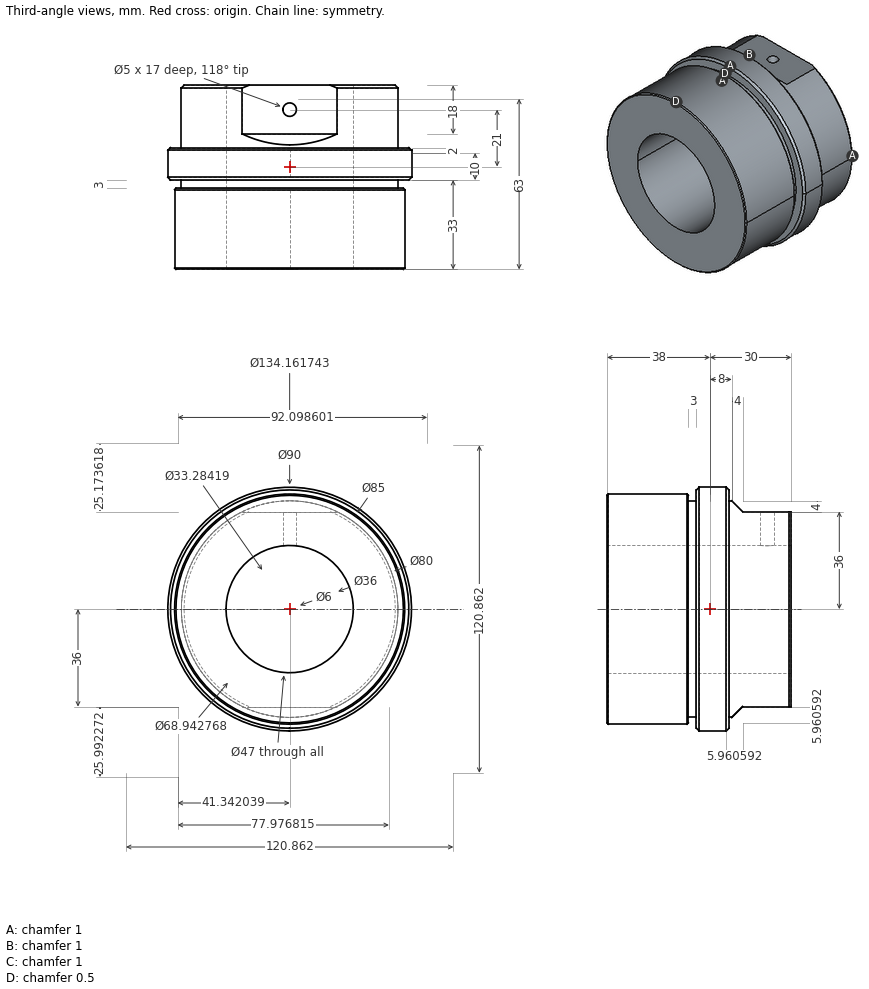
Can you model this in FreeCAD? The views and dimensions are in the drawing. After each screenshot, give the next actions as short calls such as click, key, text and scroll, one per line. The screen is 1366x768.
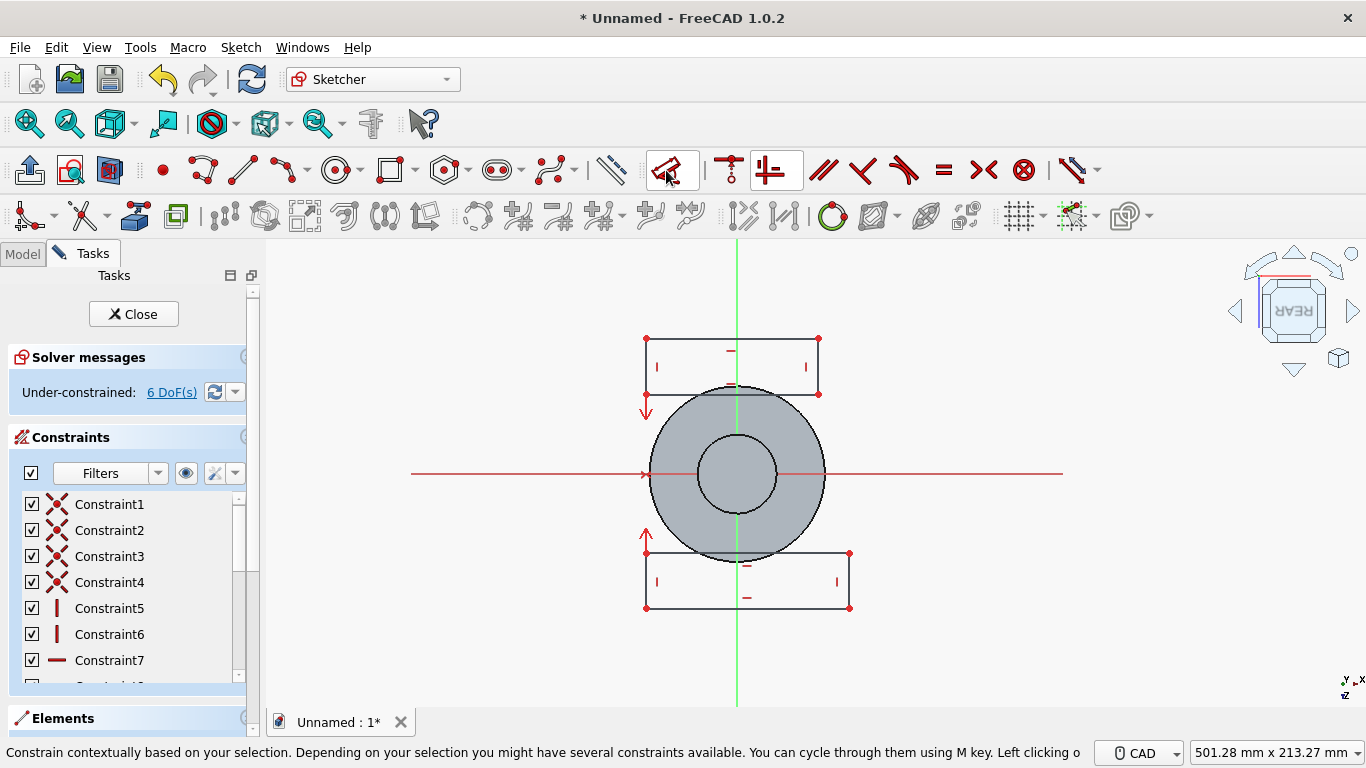
click(646, 395)
click(612, 435)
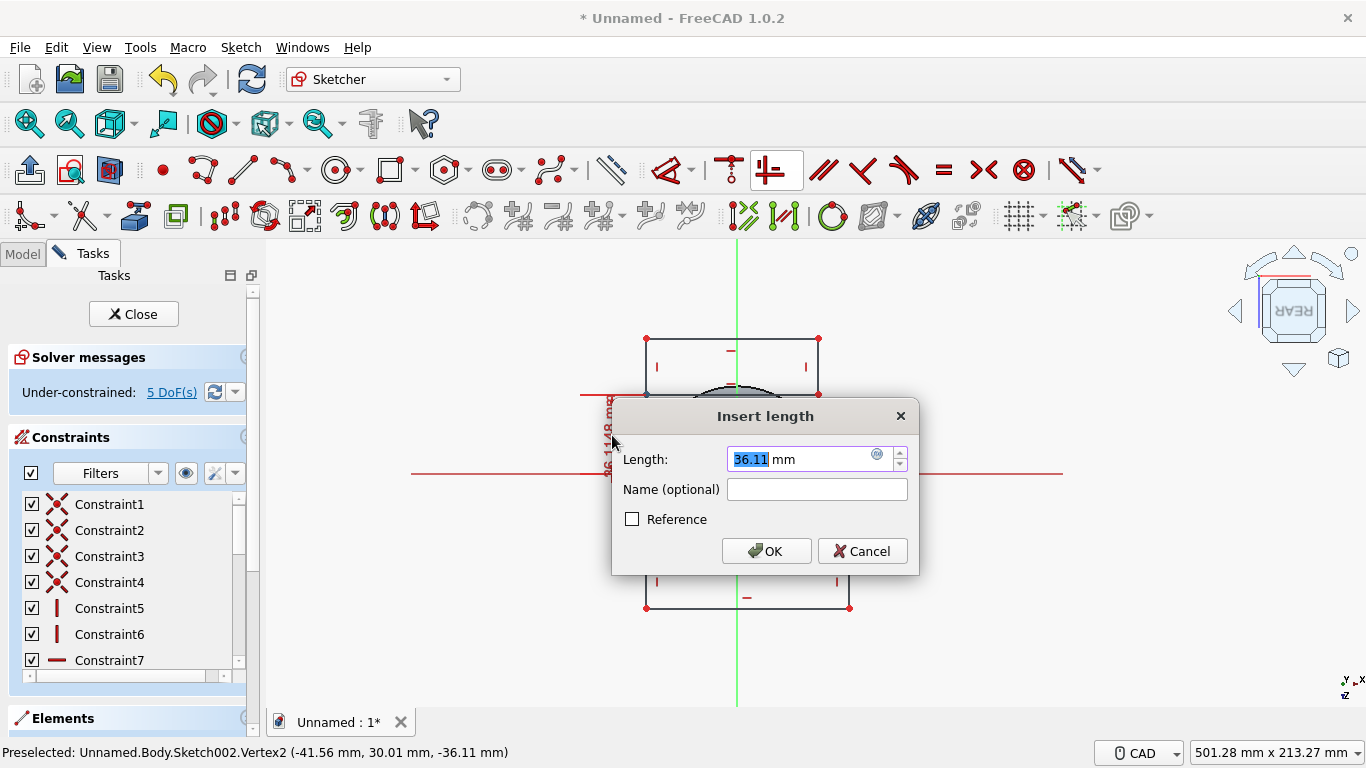
text(36)
key(Return)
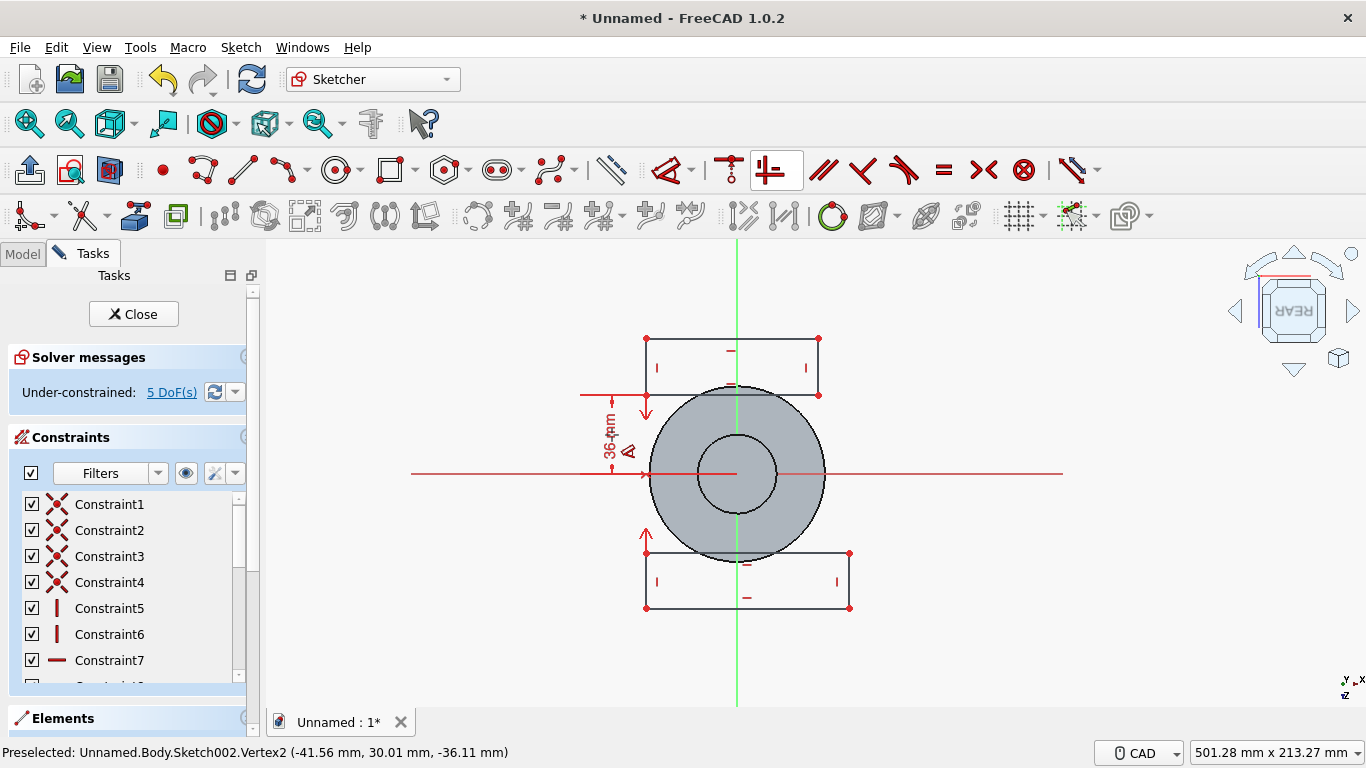
click(646, 356)
click(612, 367)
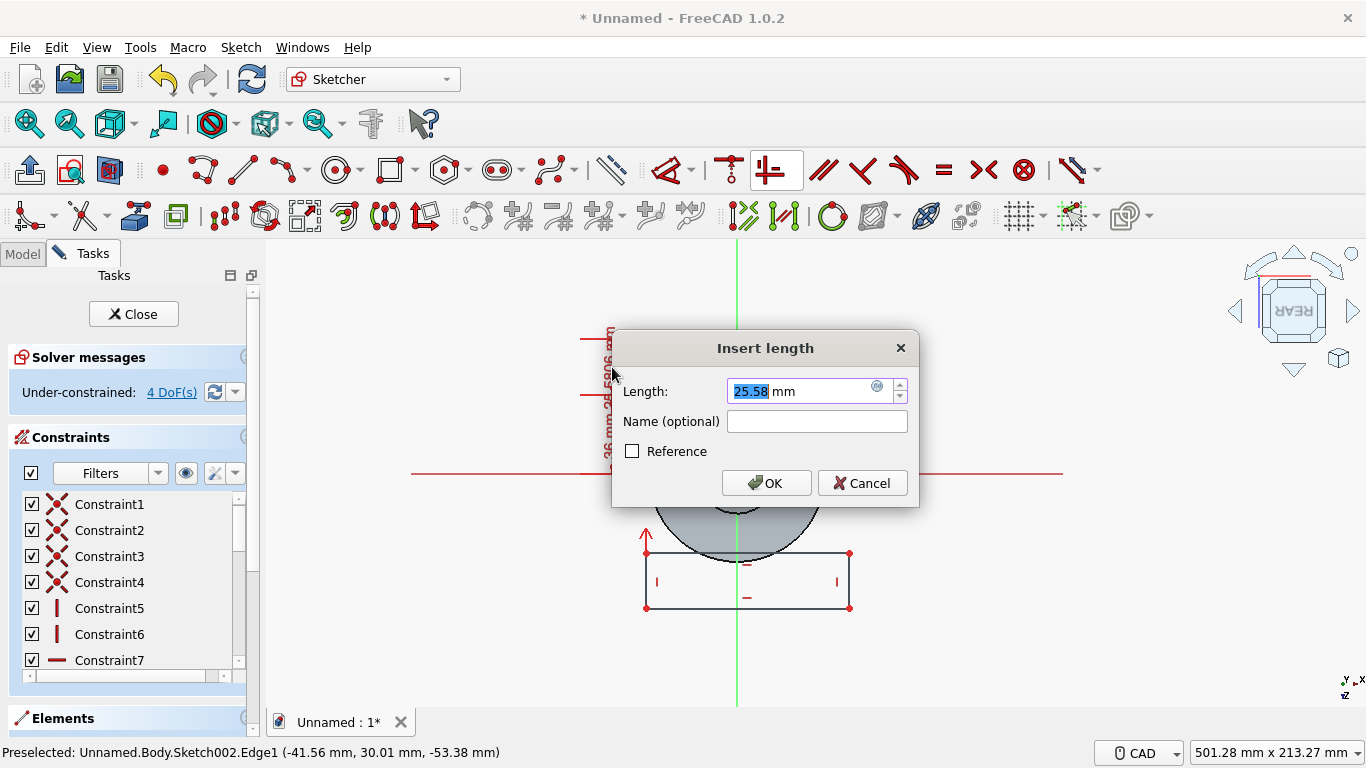
text(25.992272)
key(Return)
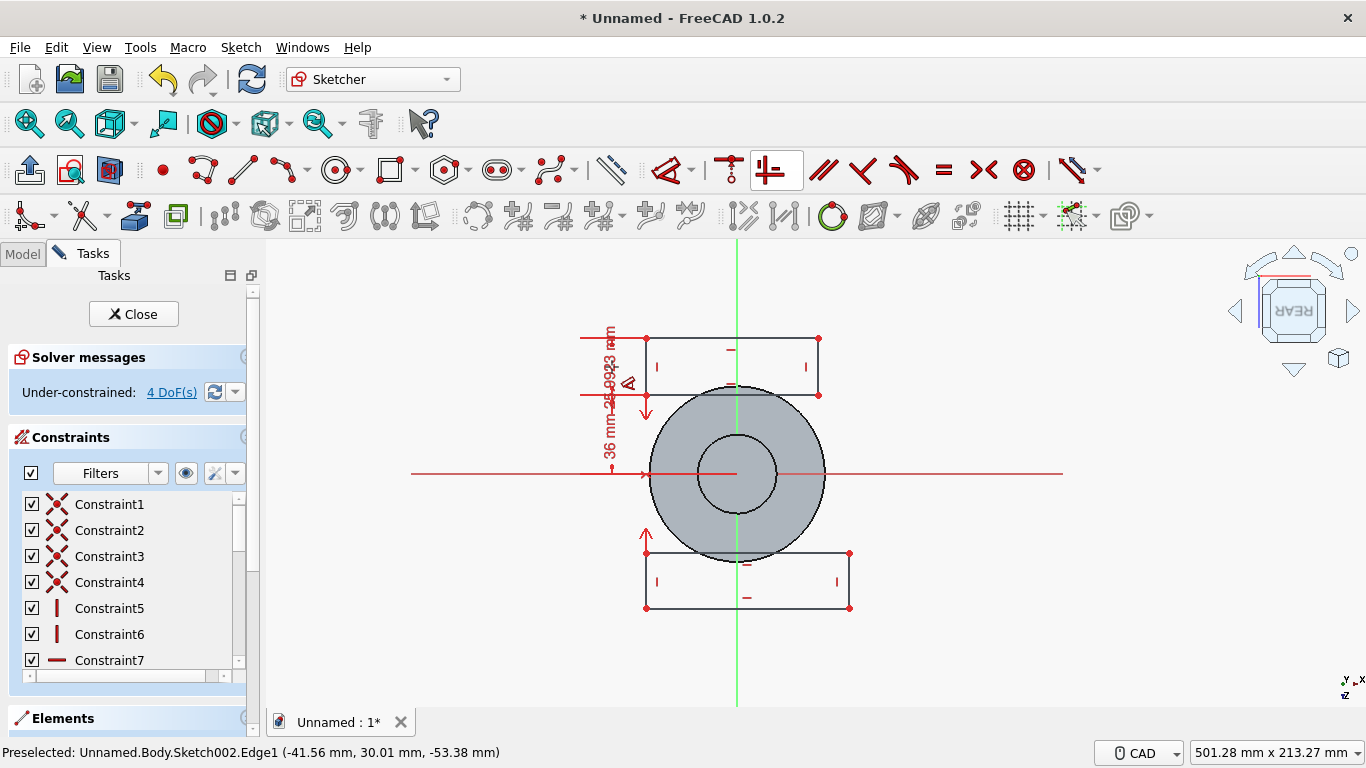
click(698, 395)
click(692, 361)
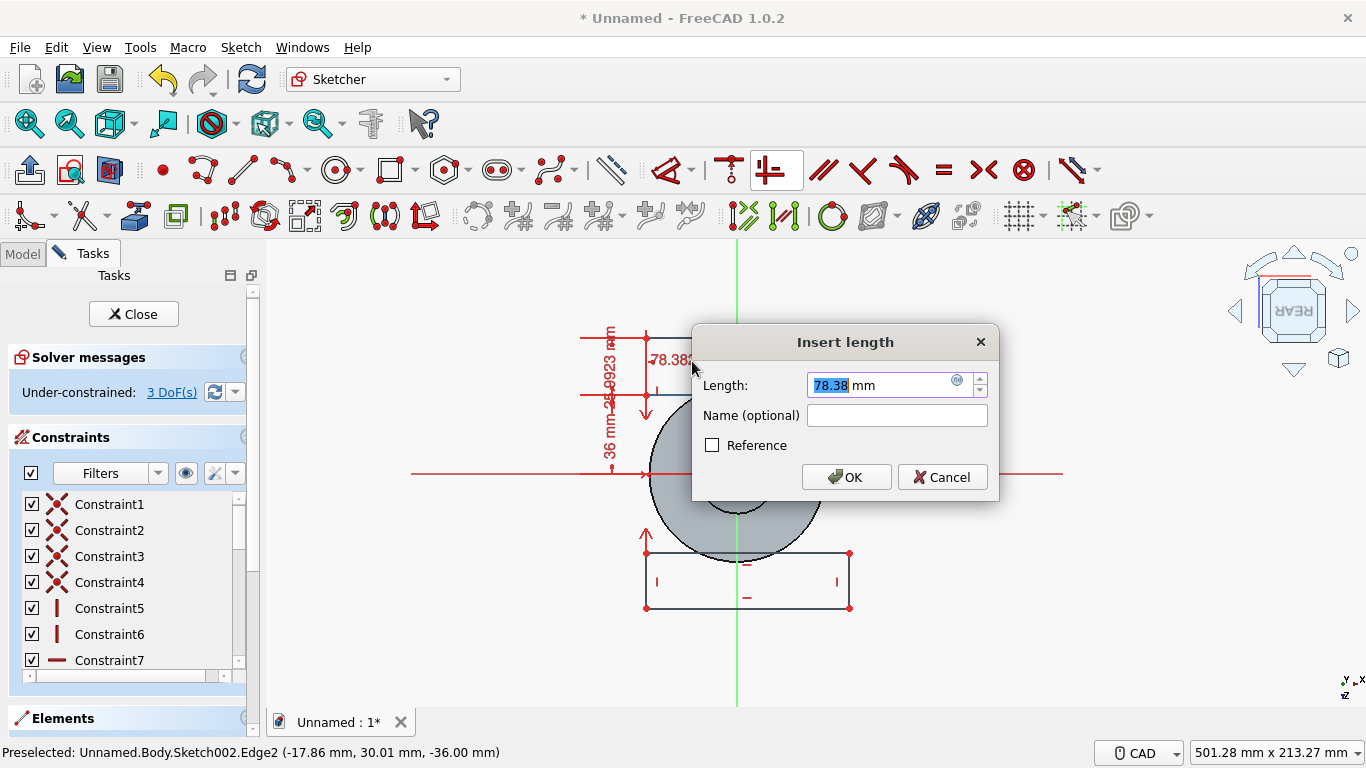
text(77.976815)
key(Return)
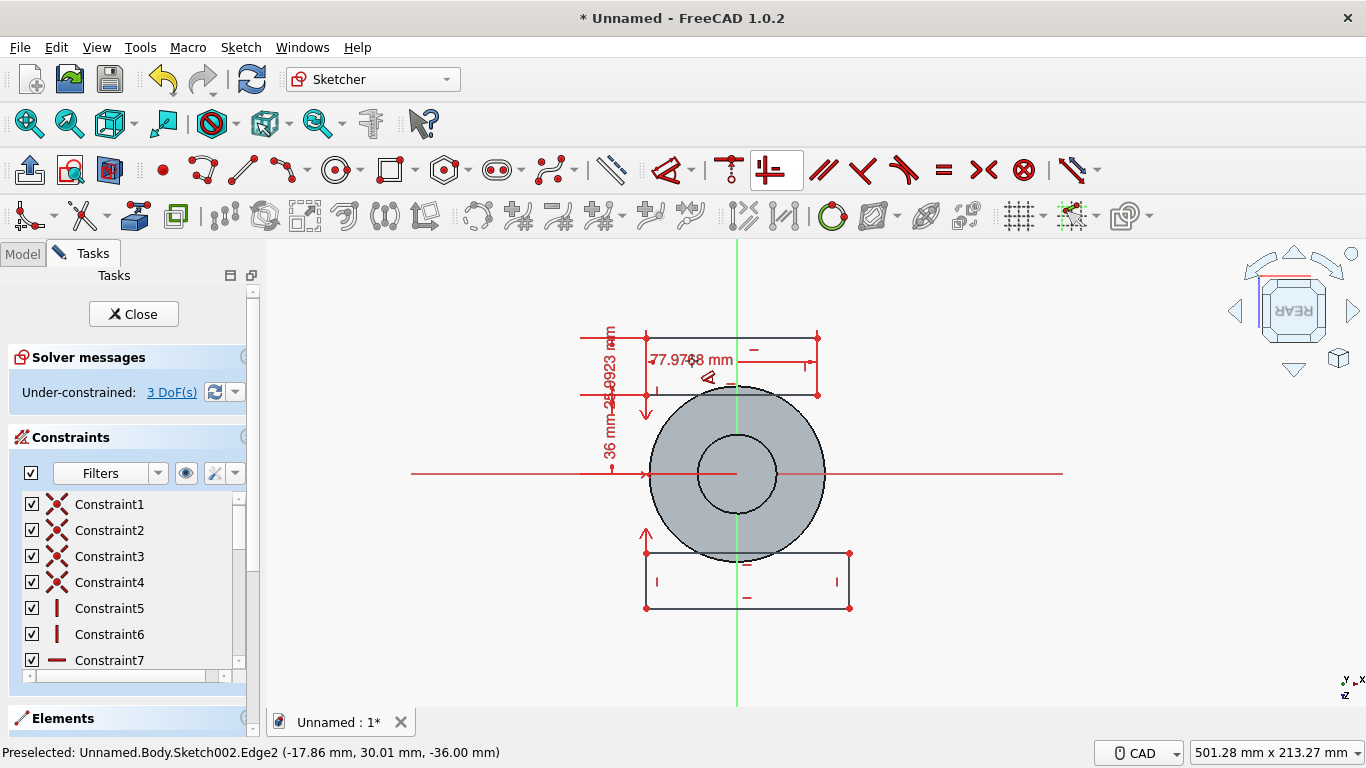
click(646, 570)
click(612, 581)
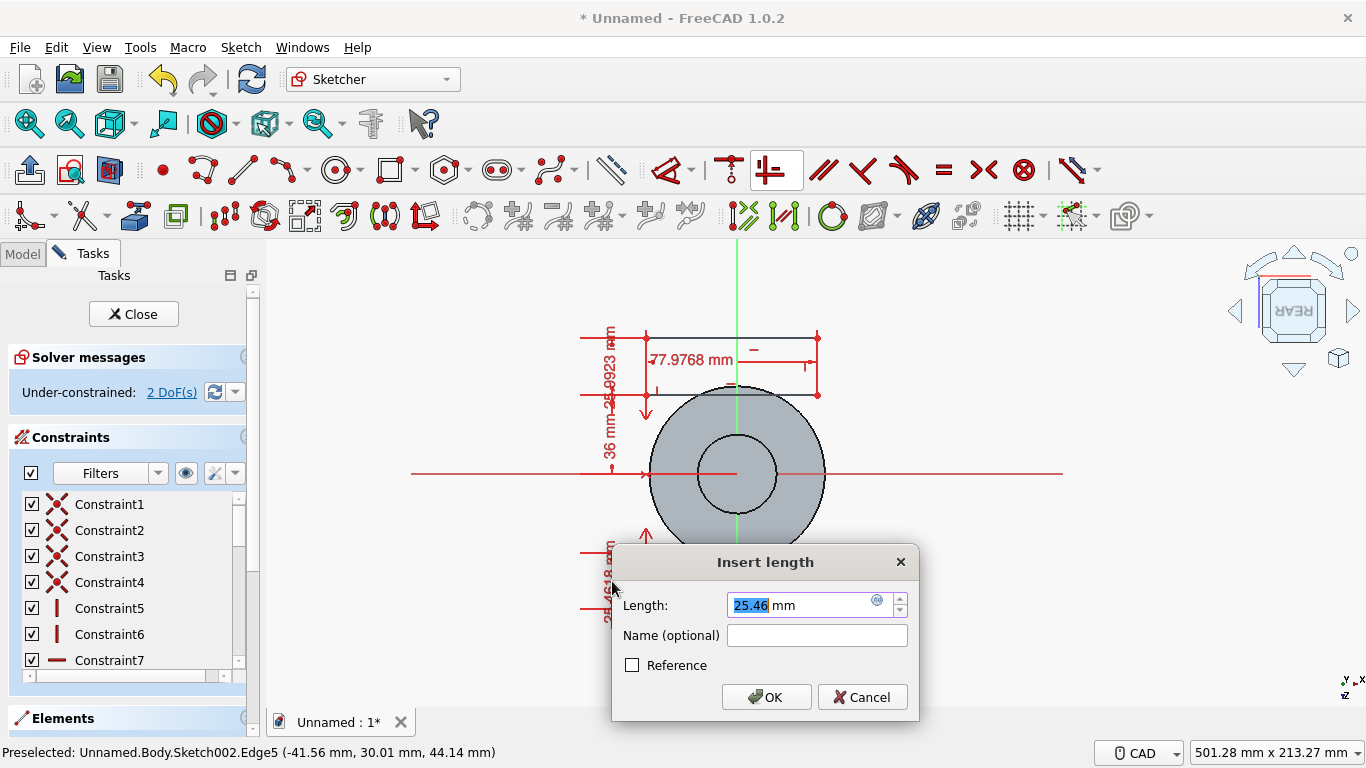
text(25.173618)
key(Return)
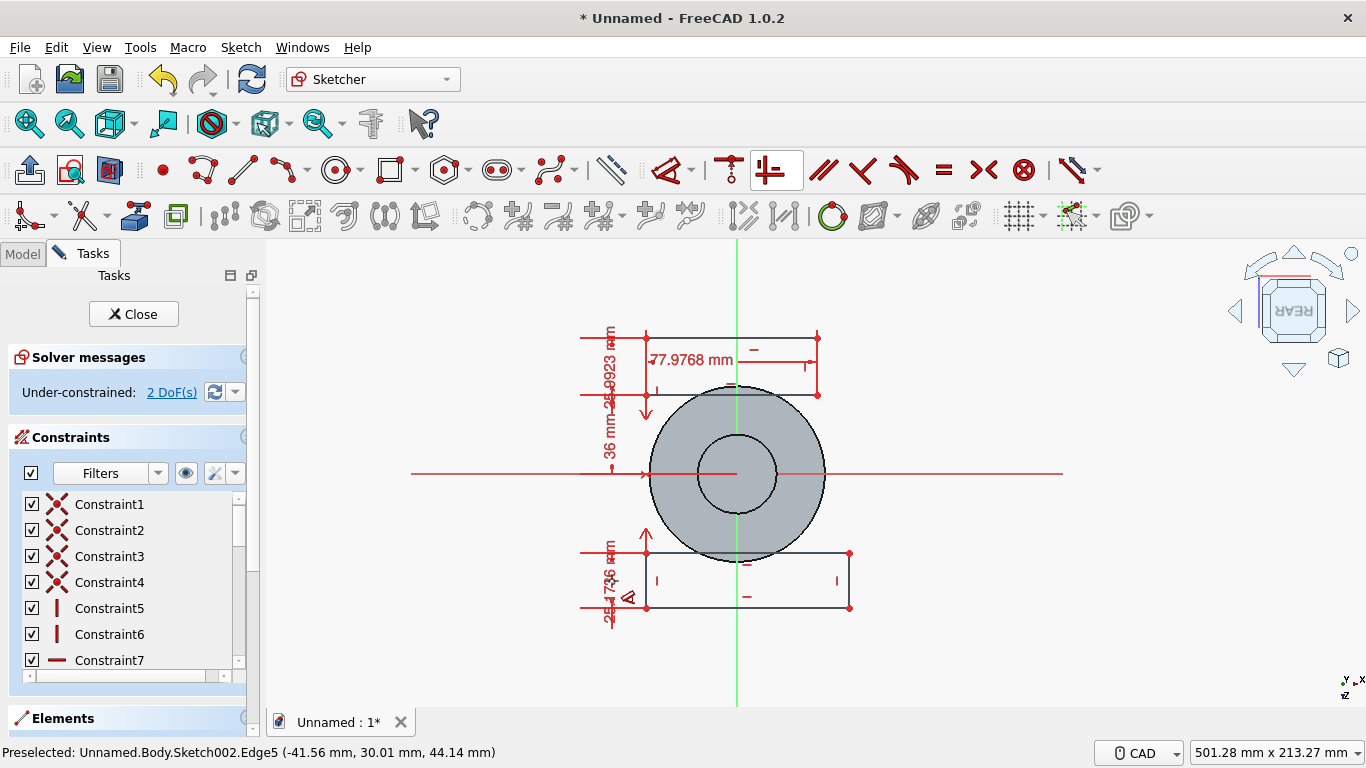
click(707, 608)
click(701, 642)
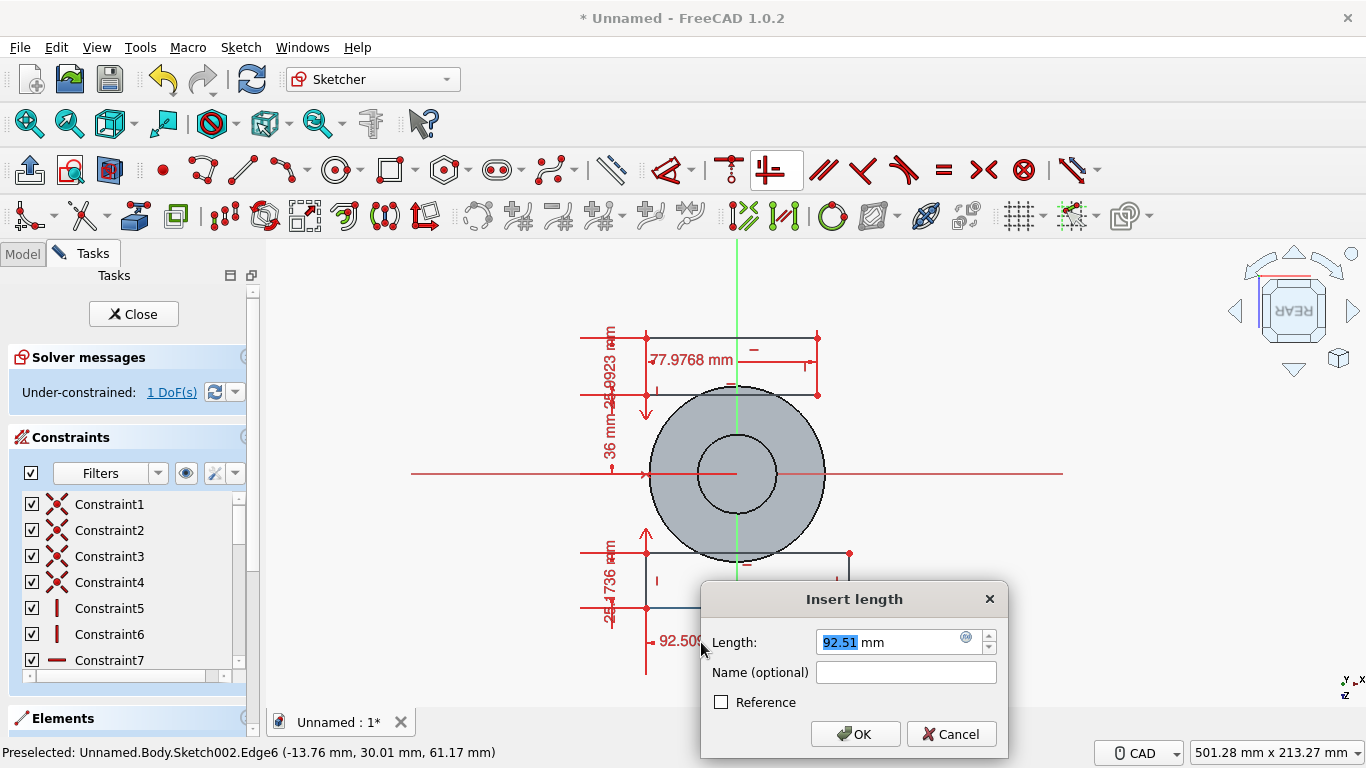
text(92.098601)
key(Return)